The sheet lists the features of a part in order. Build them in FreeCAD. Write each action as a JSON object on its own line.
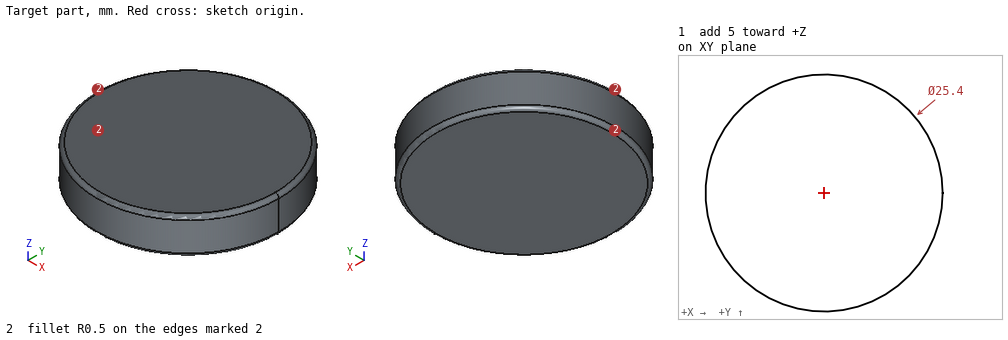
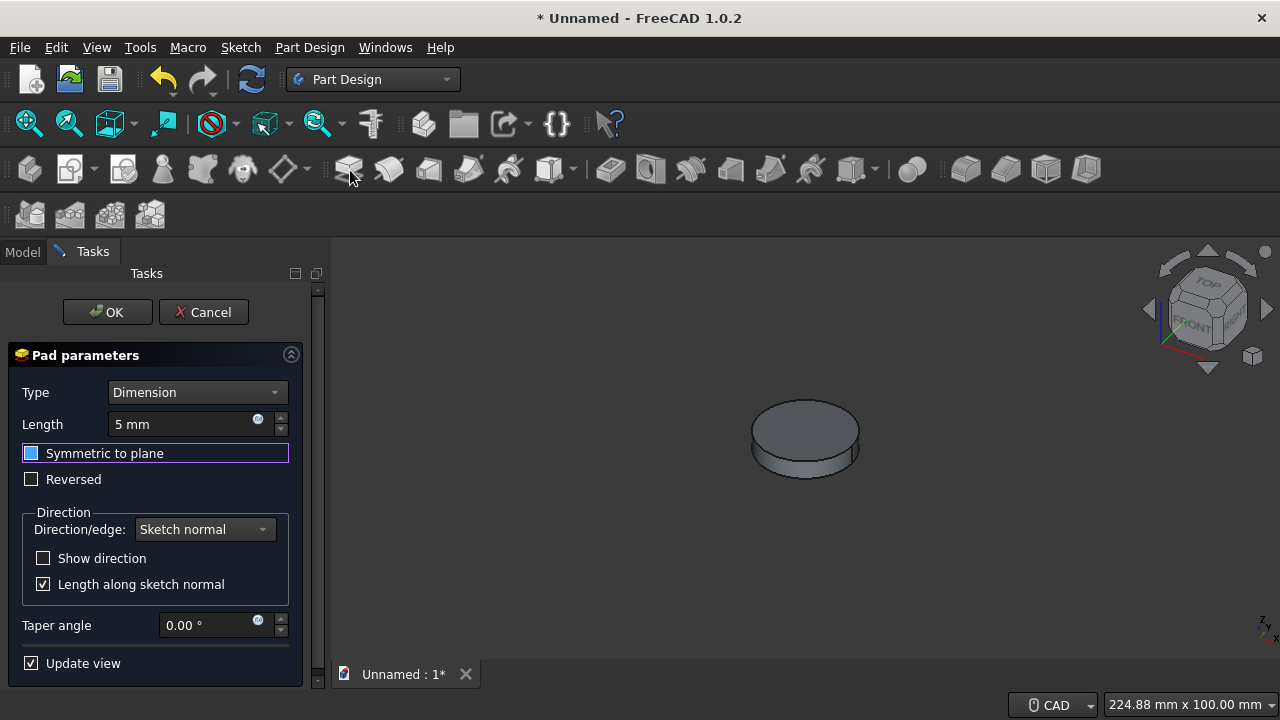
{"action": "left_click", "coordinate": [108, 312]}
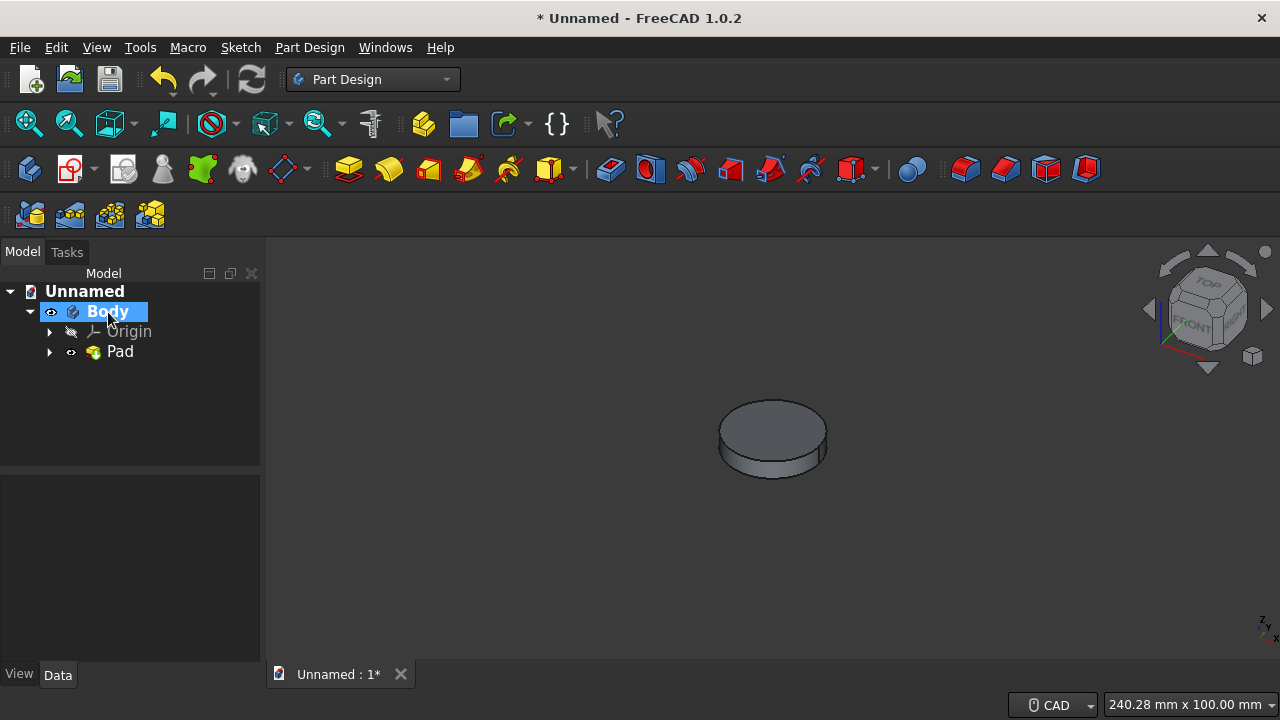
{"action": "left_click", "coordinate": [30, 124]}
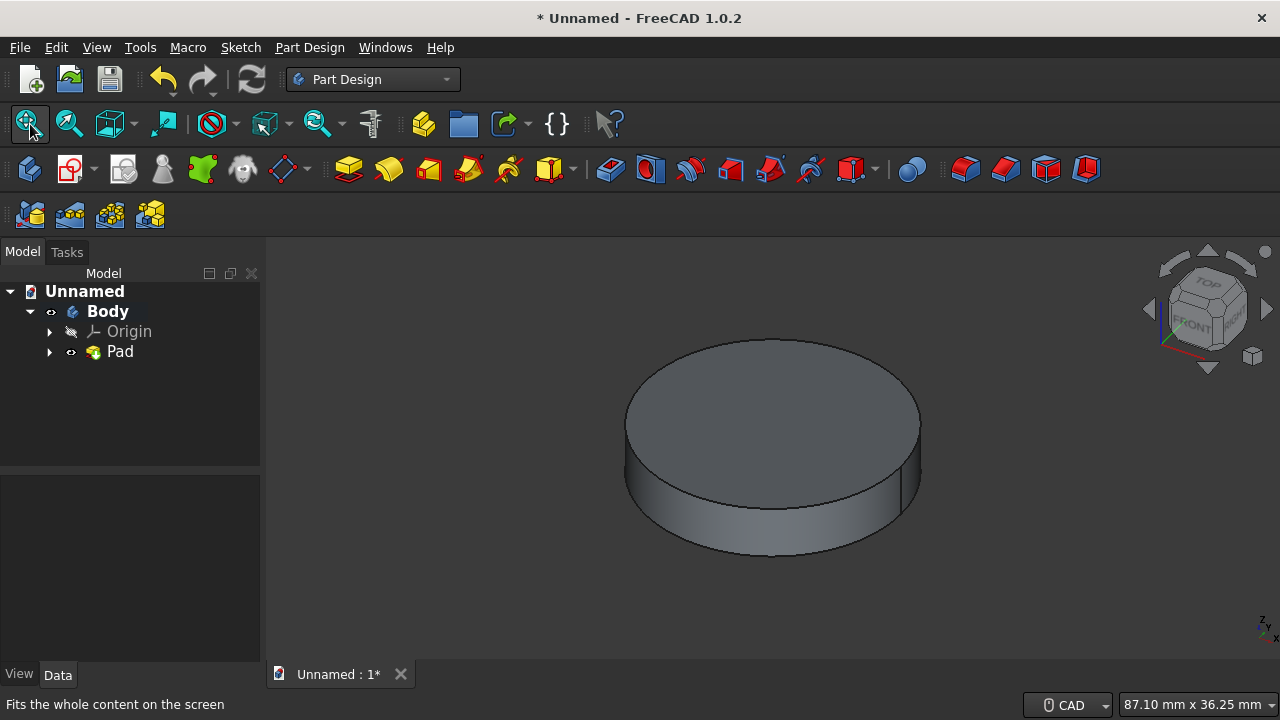
{"action": "left_click", "coordinate": [626, 432]}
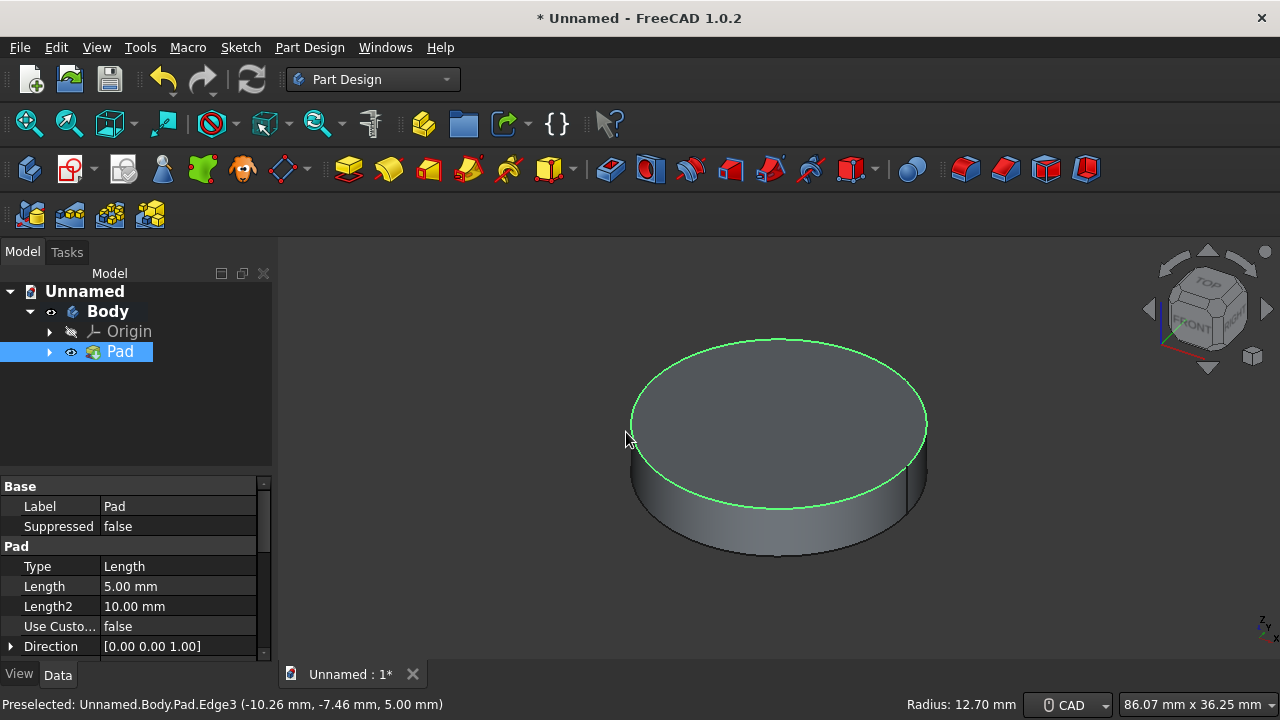
{"action": "key", "text": "0"}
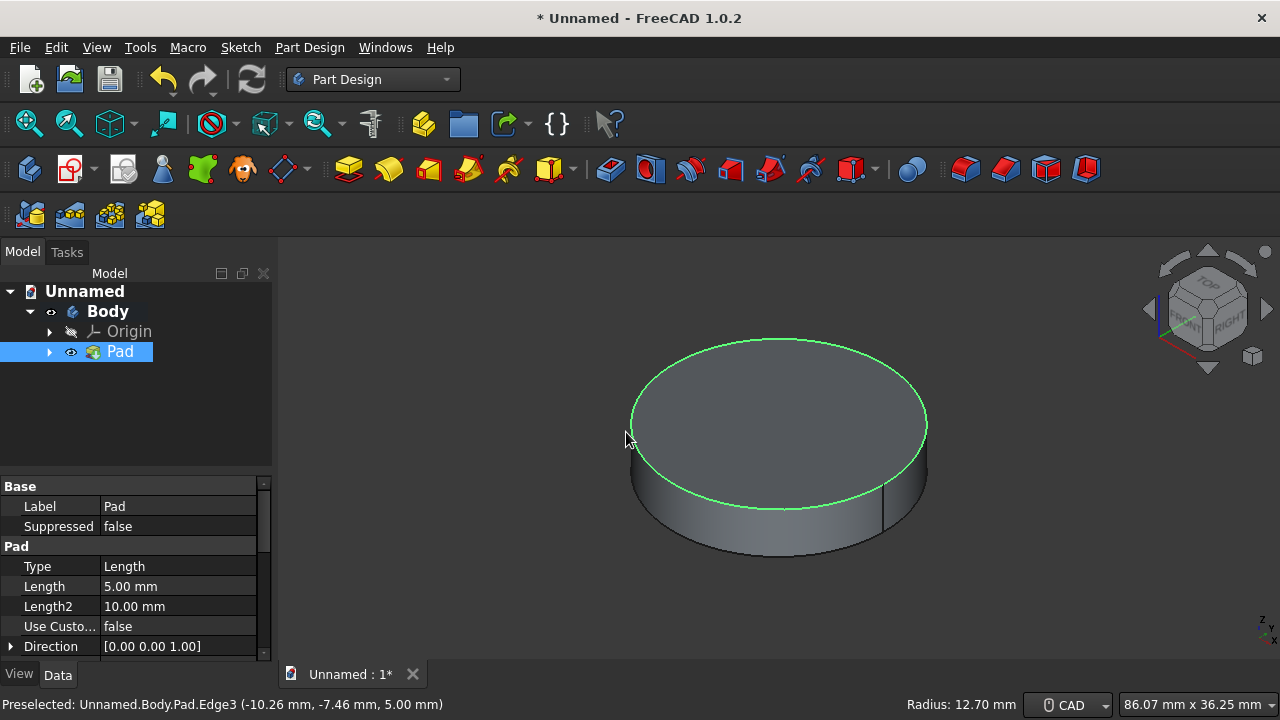
{"action": "key", "text": "2"}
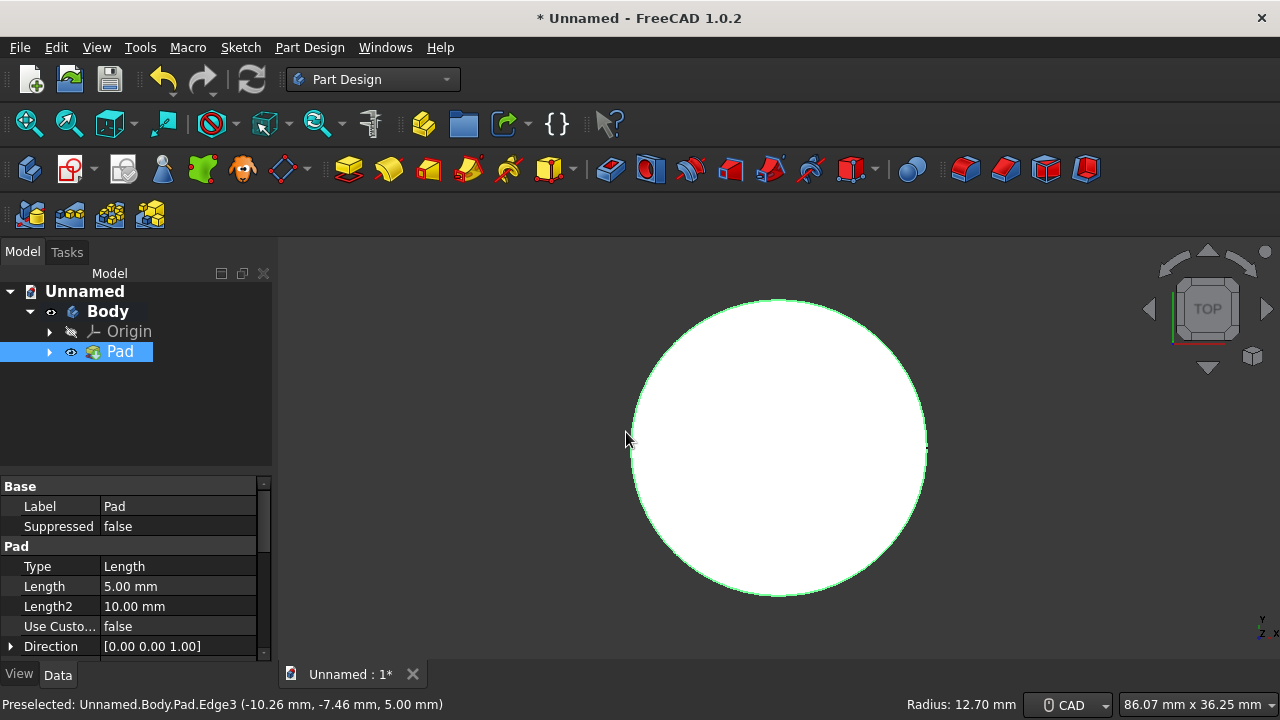
{"action": "key", "text": "1"}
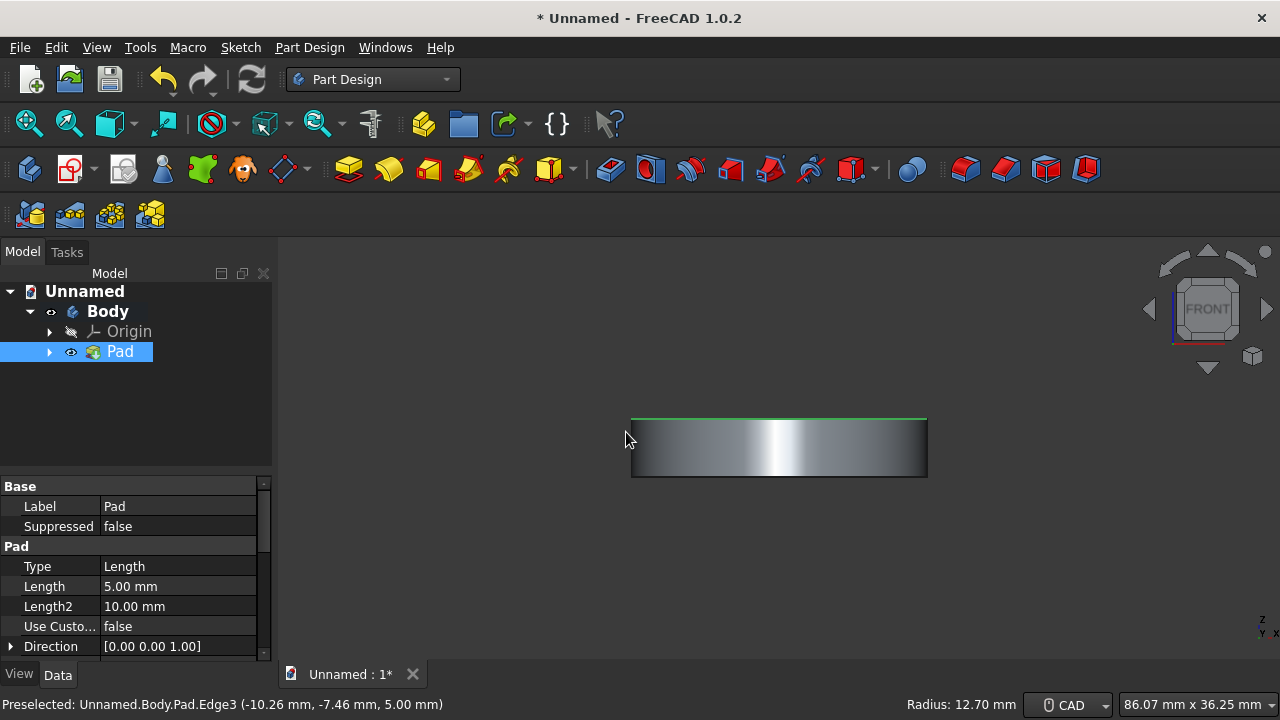
{"action": "left_click", "coordinate": [30, 124]}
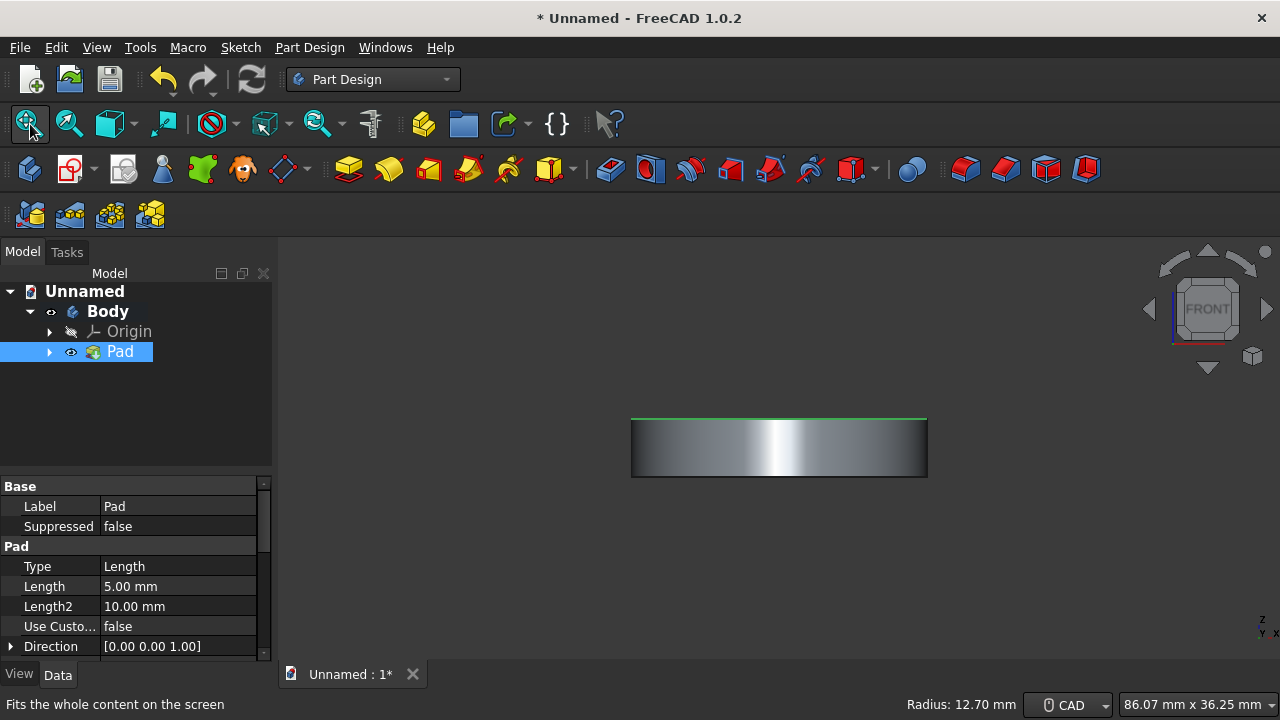
{"action": "left_click", "coordinate": [659, 476], "text": "ctrl"}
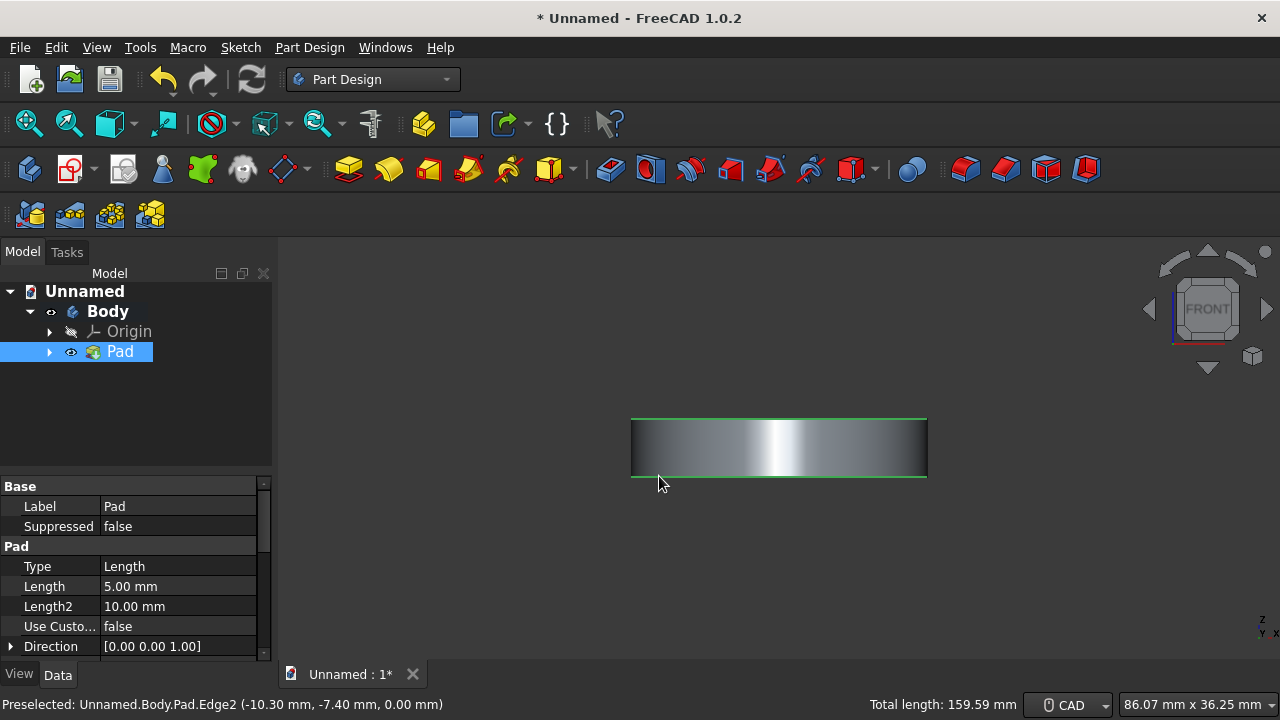
{"action": "left_click", "coordinate": [966, 170]}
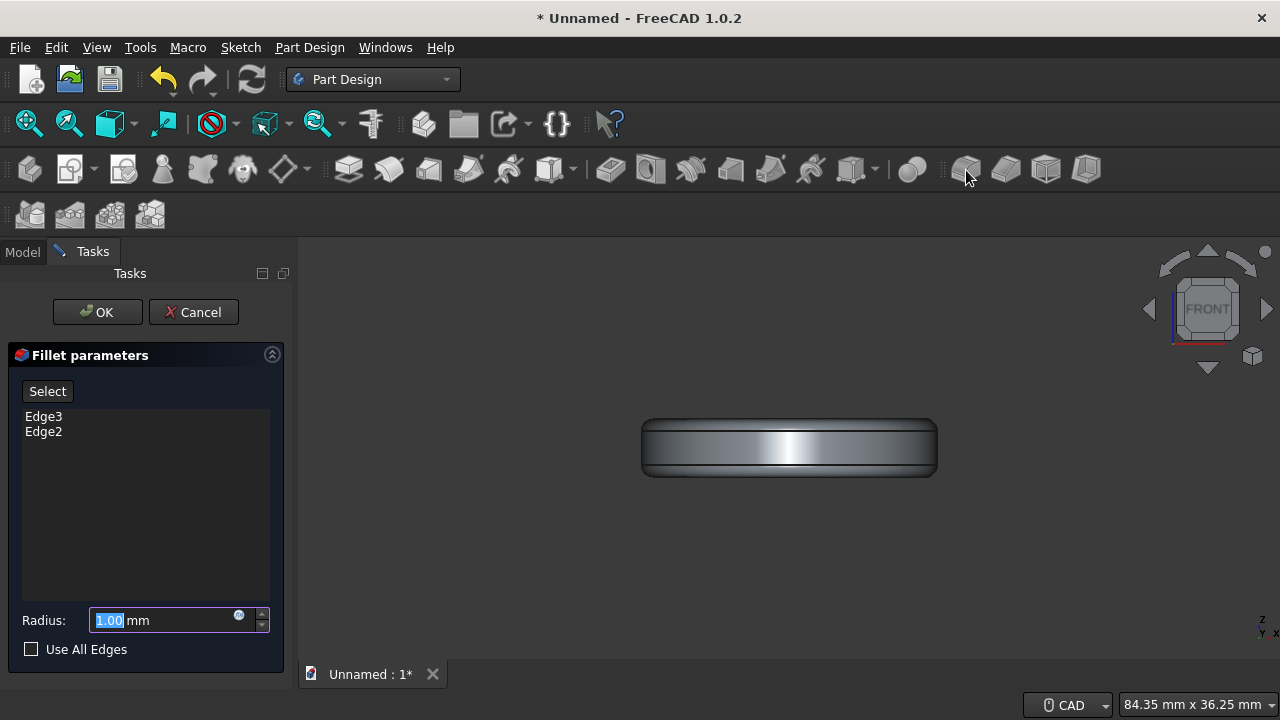
{"action": "type", "text": "0.5"}
{"action": "key", "text": "Tab"}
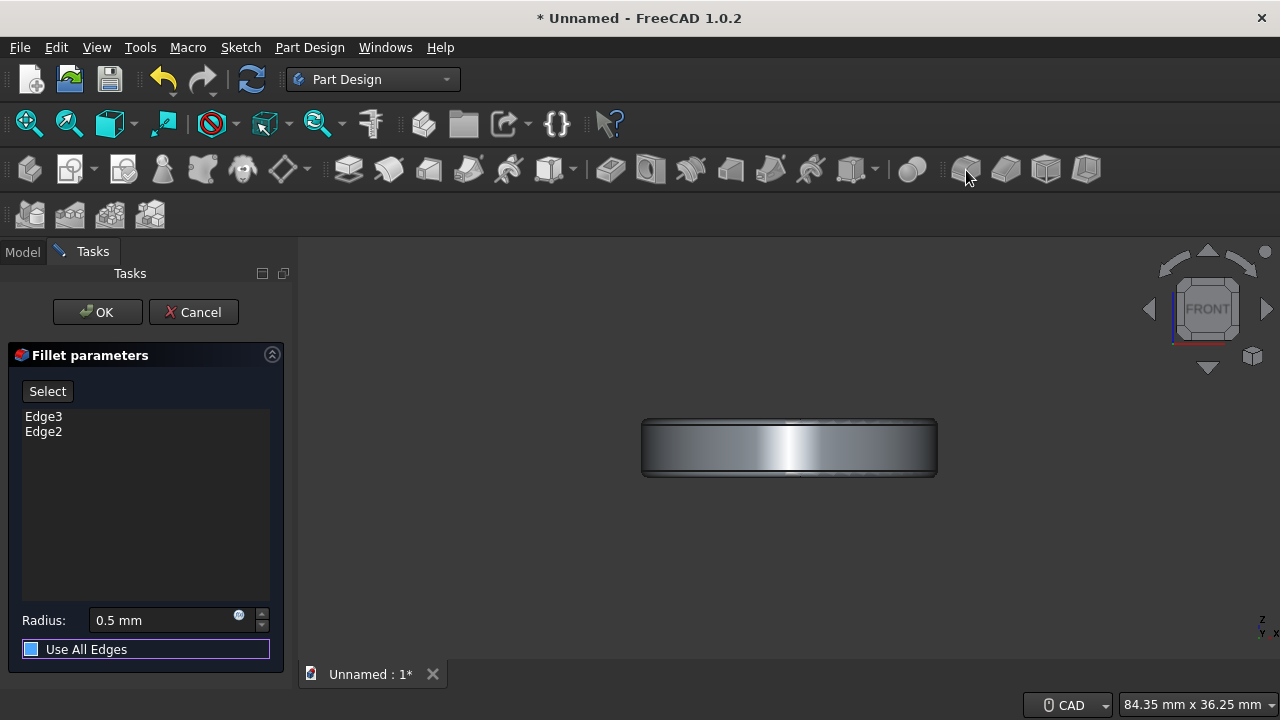
{"action": "left_click", "coordinate": [98, 312]}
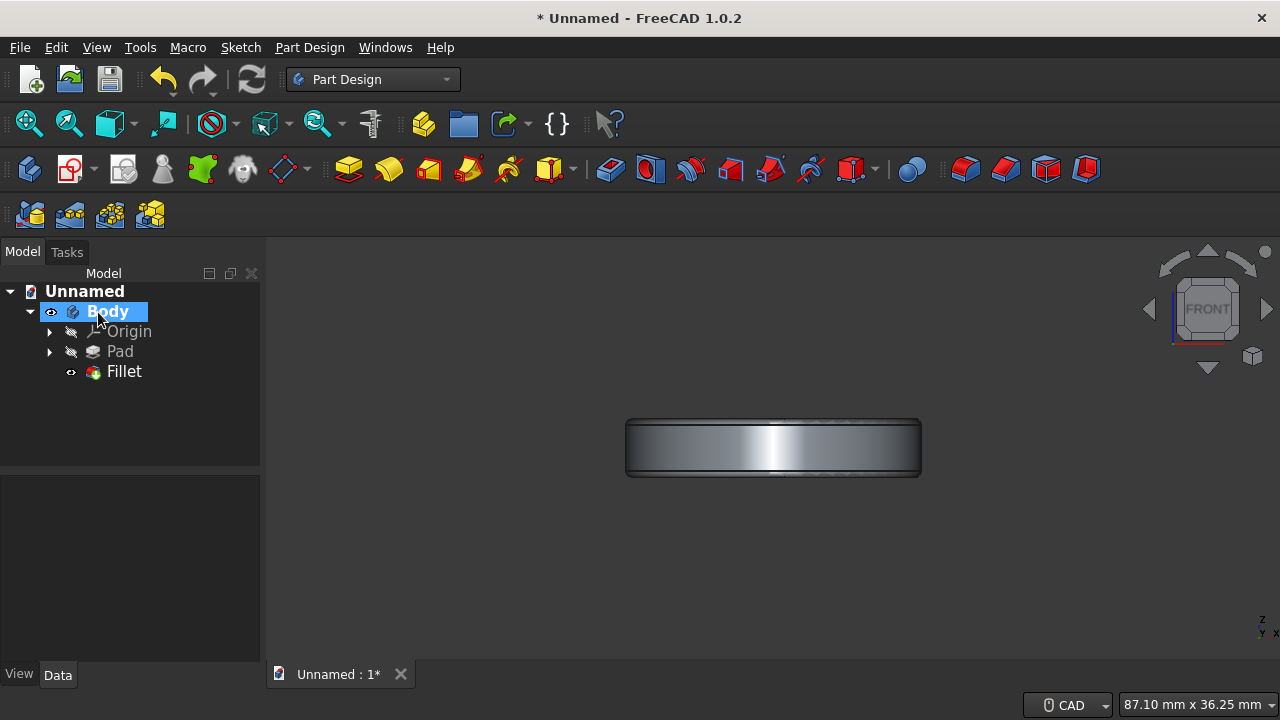
{"action": "key", "text": "0"}